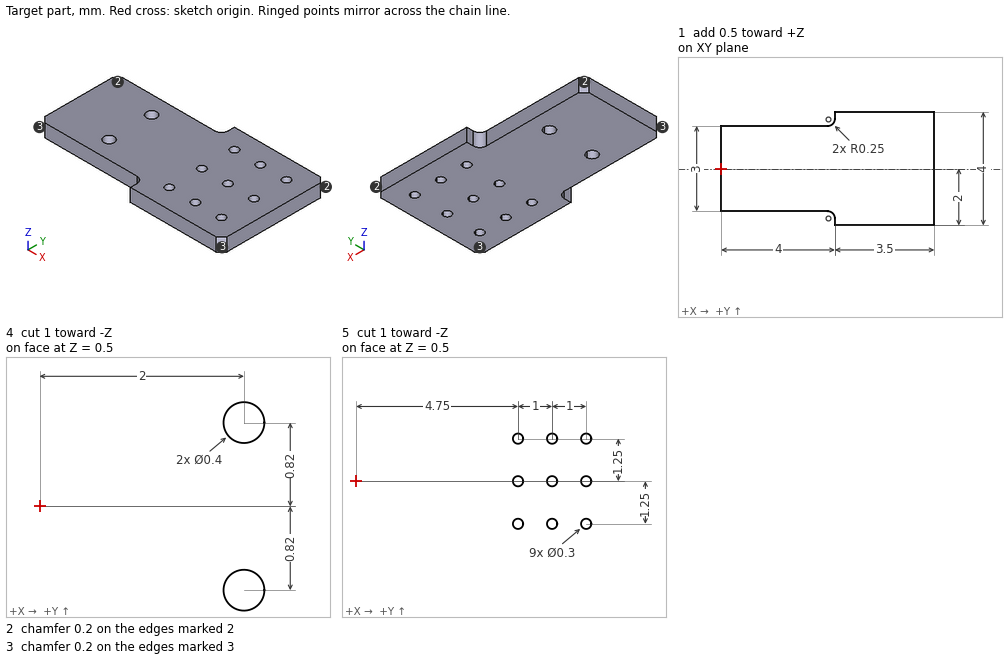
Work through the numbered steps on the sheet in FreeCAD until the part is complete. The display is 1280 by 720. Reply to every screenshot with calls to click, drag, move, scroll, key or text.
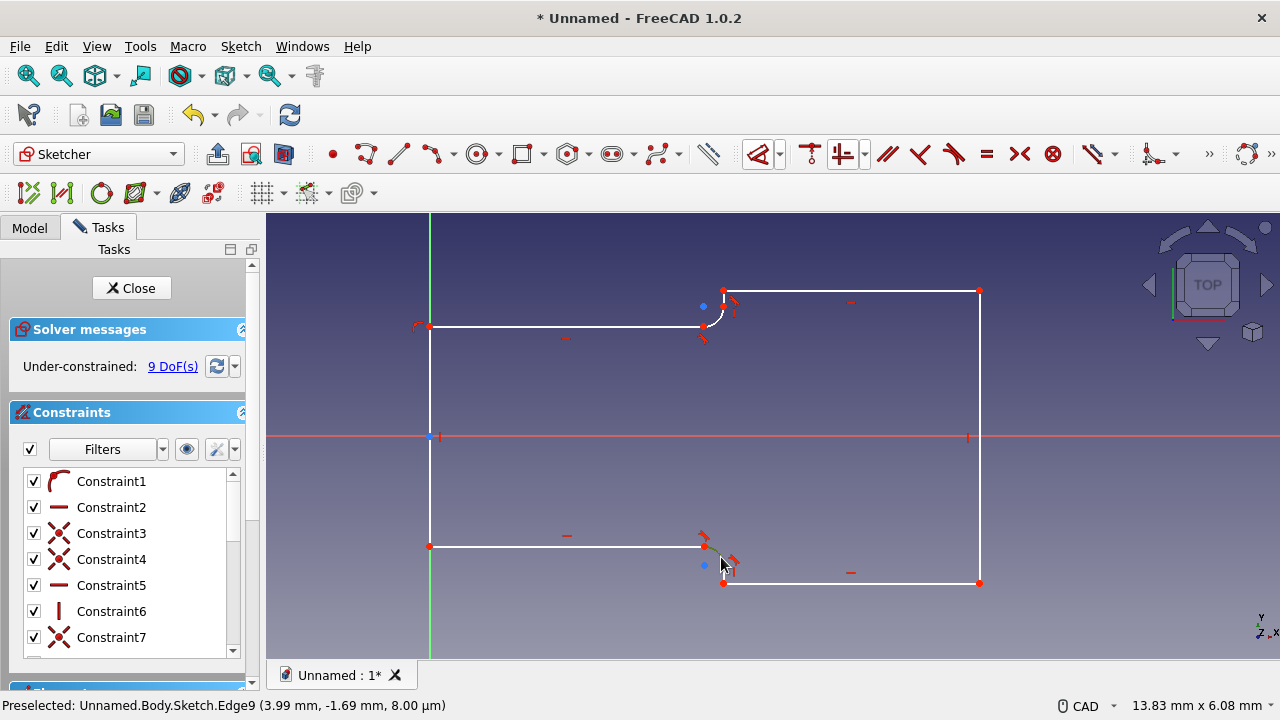
scroll(713, 325, up, 2)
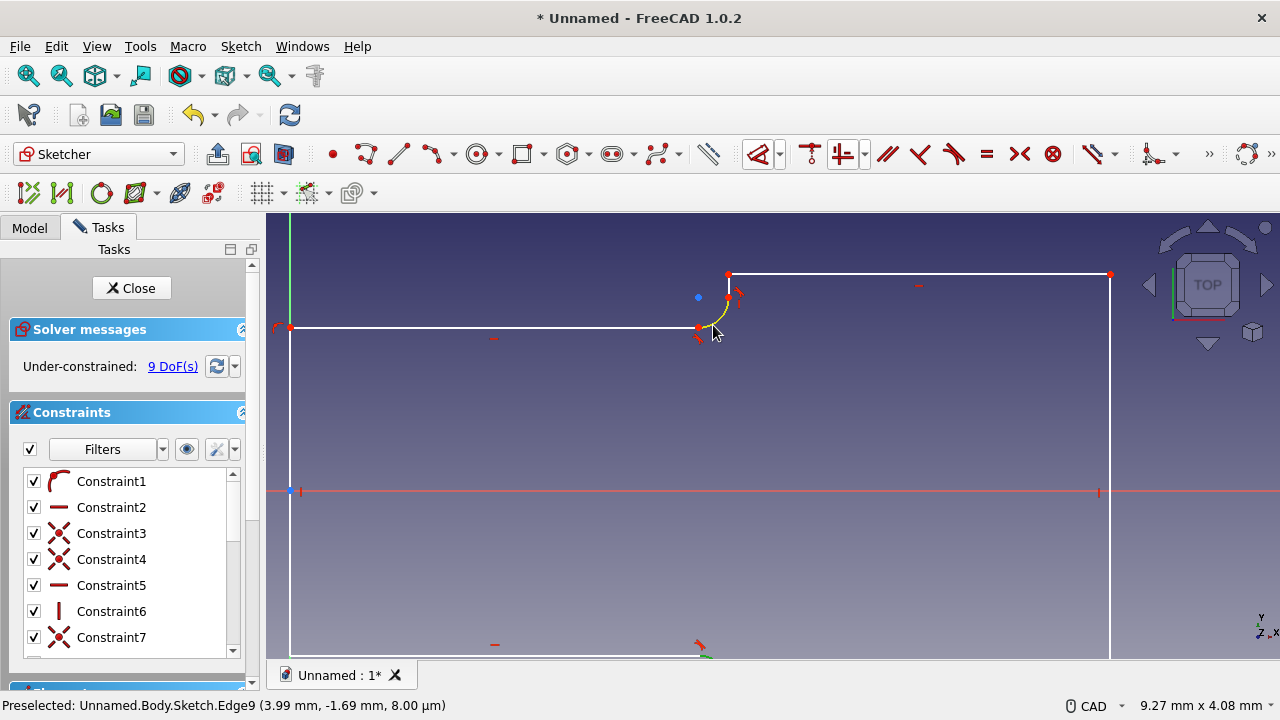
click(712, 325)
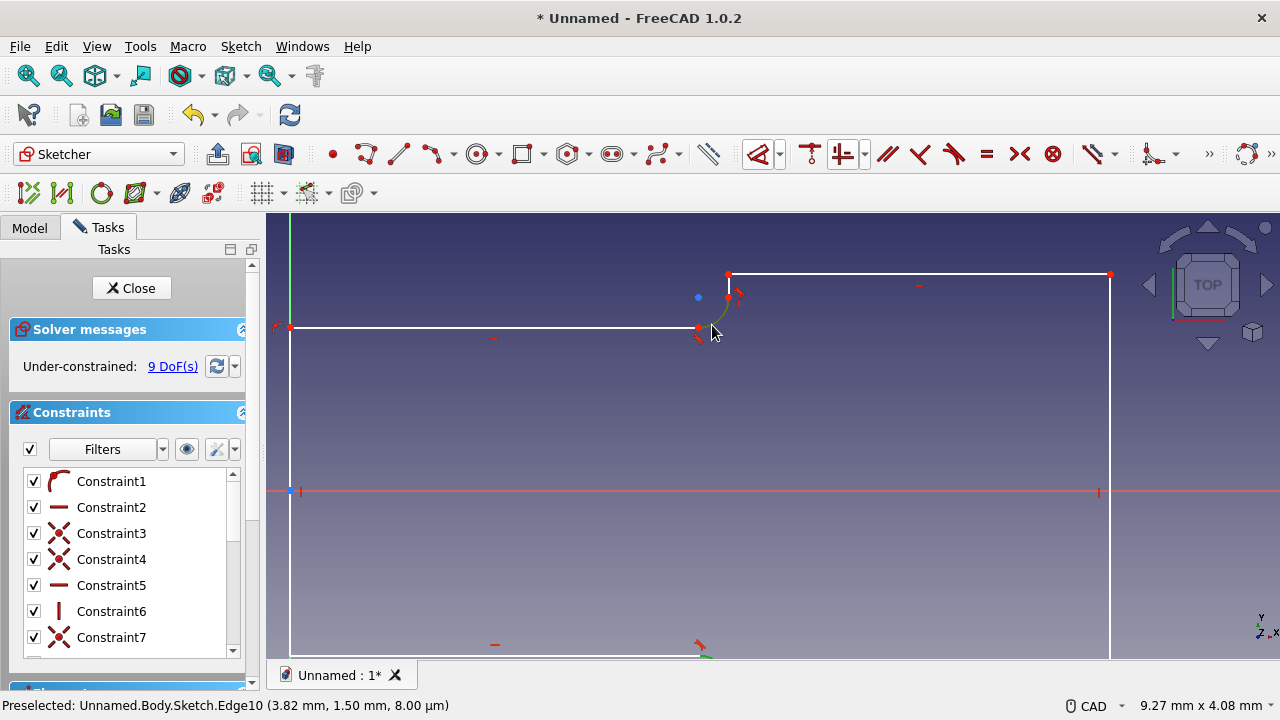
key(e)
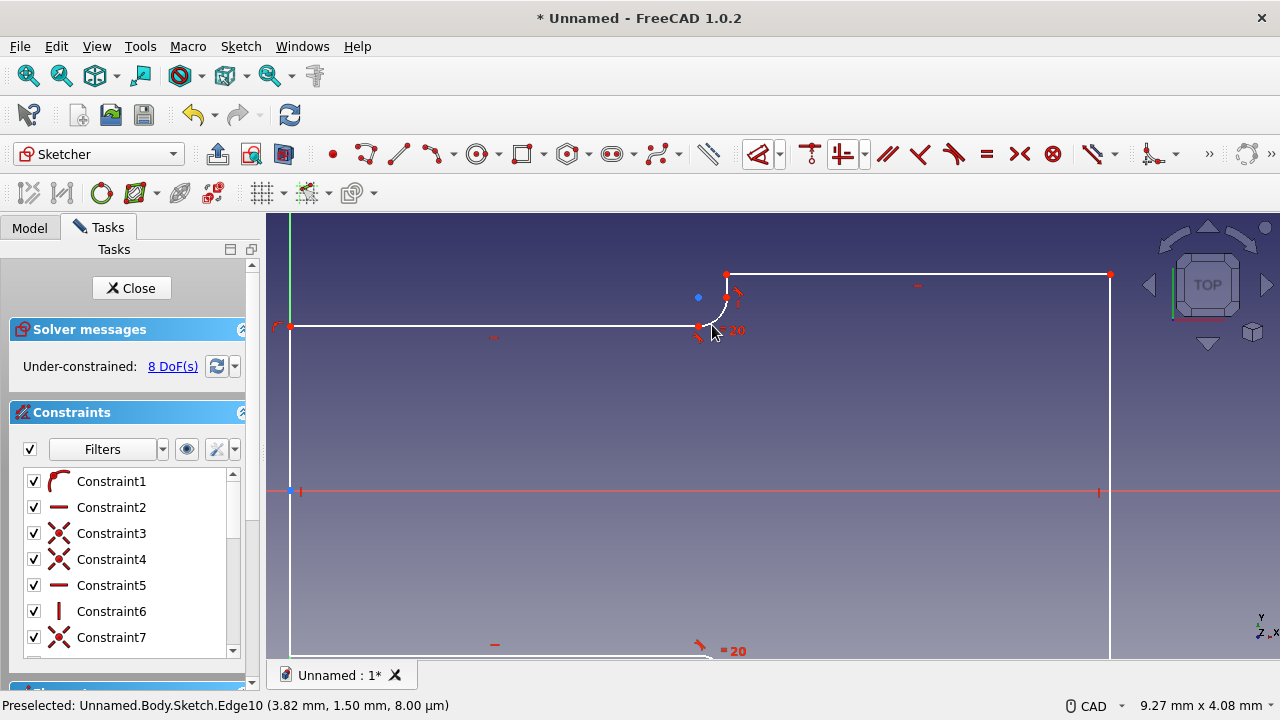
scroll(713, 325, down, 2)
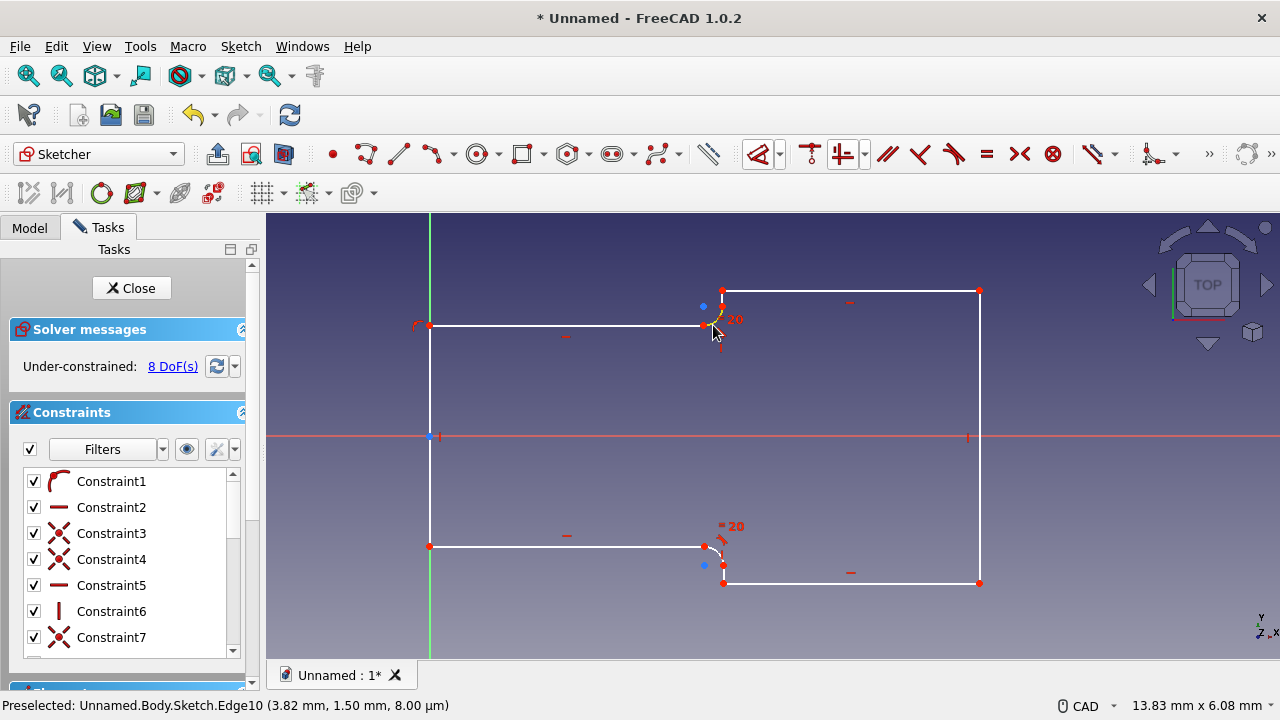
click(705, 566)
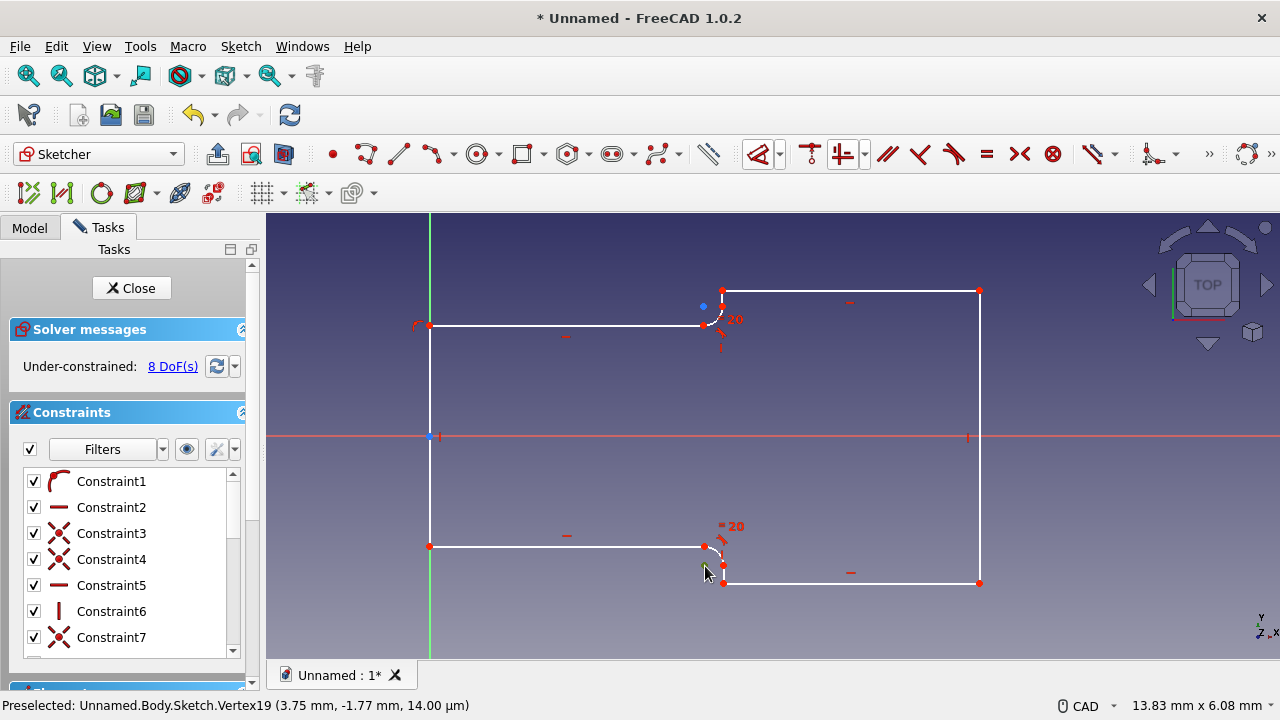
click(703, 307)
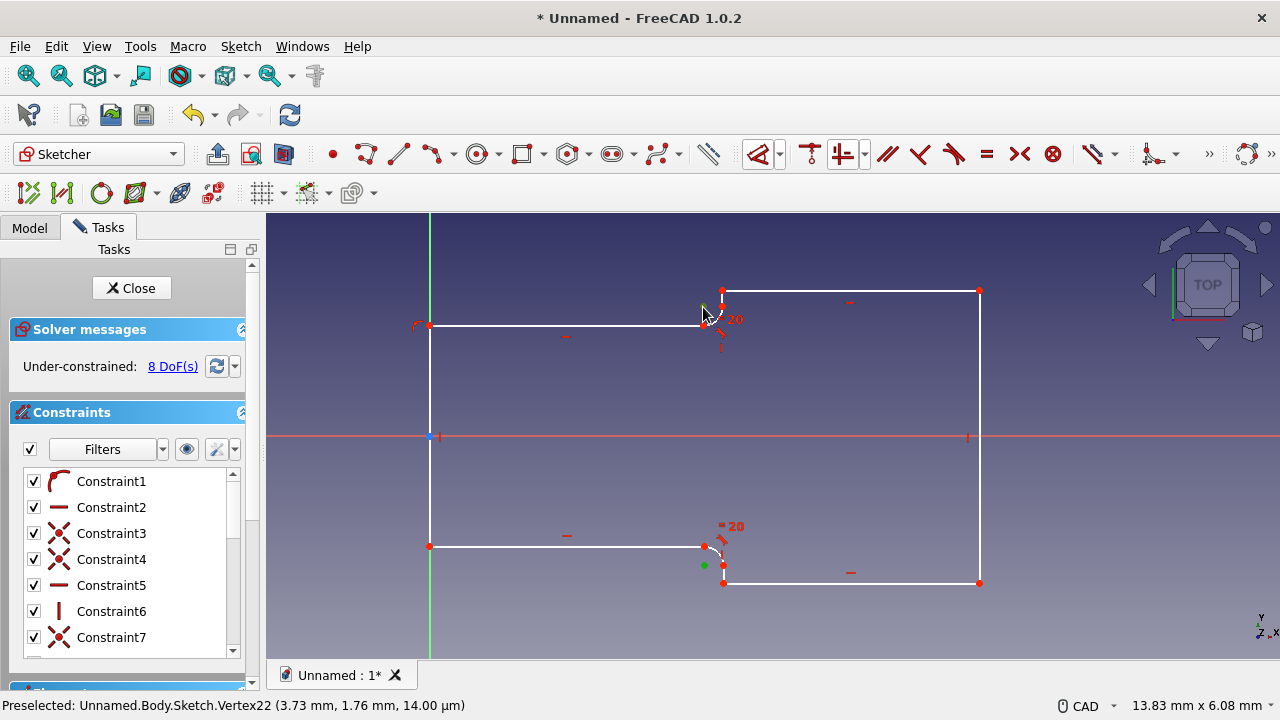
click(353, 436)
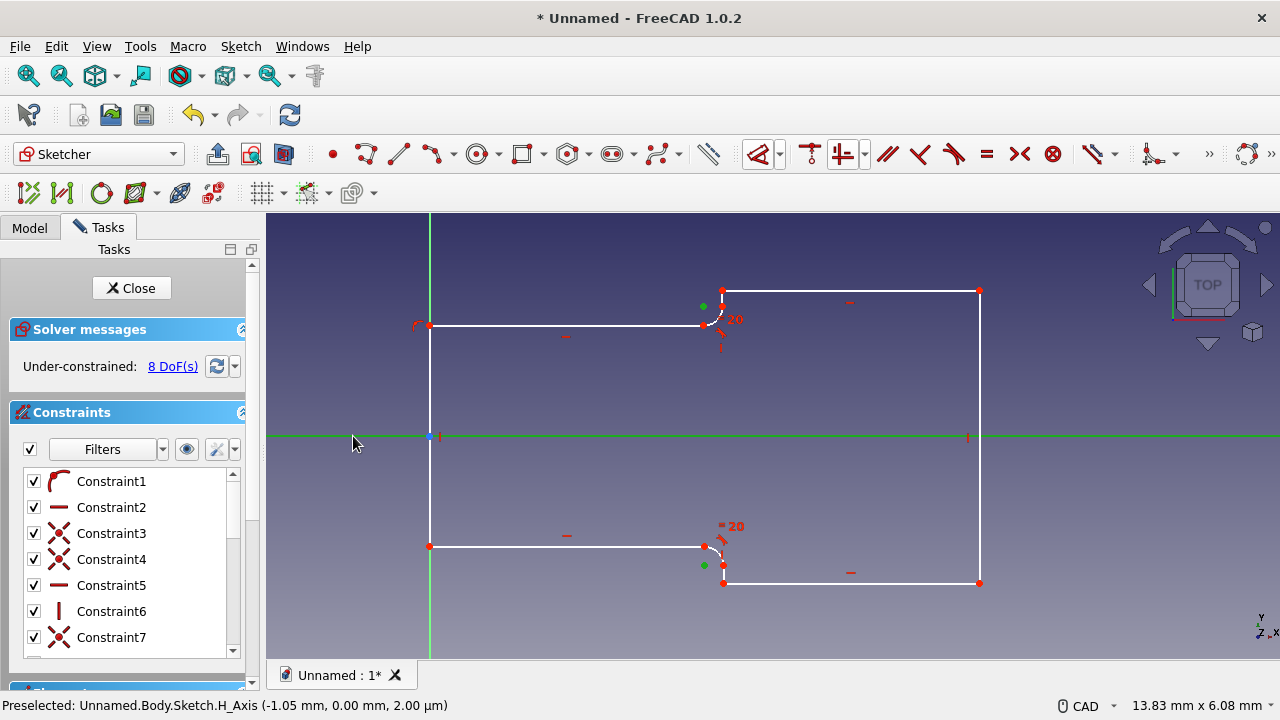
key(s)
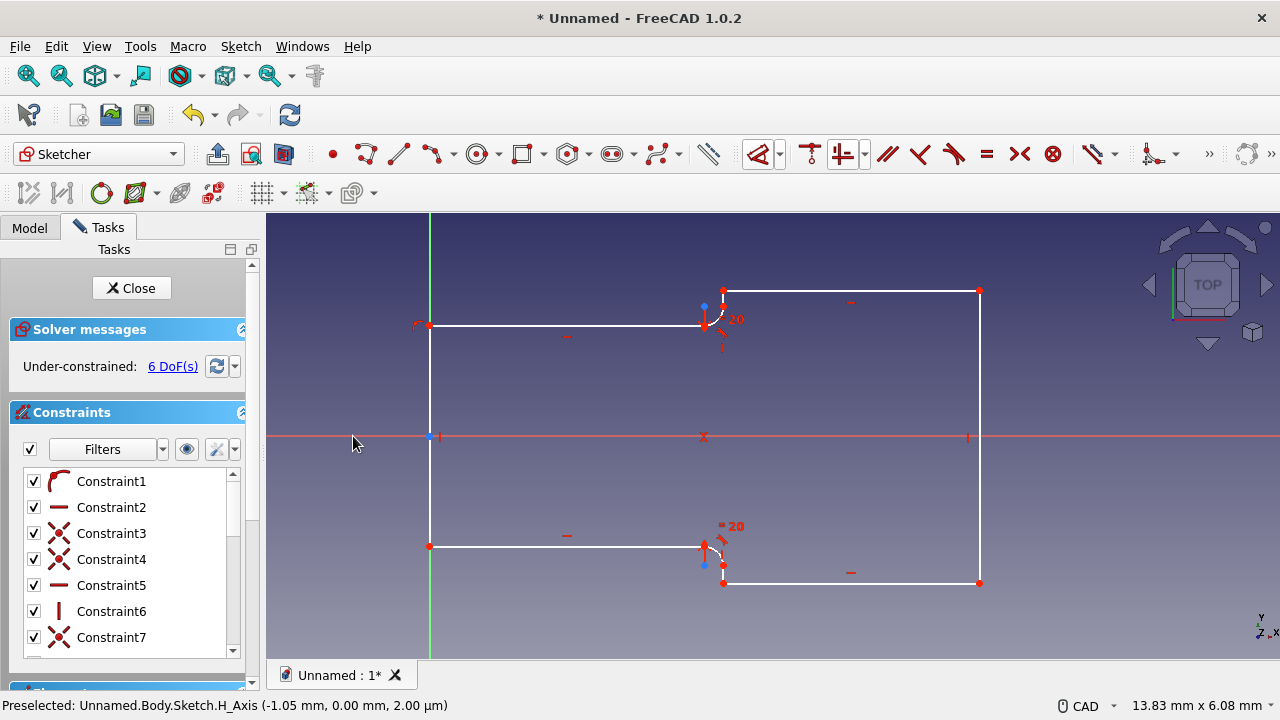
key(d)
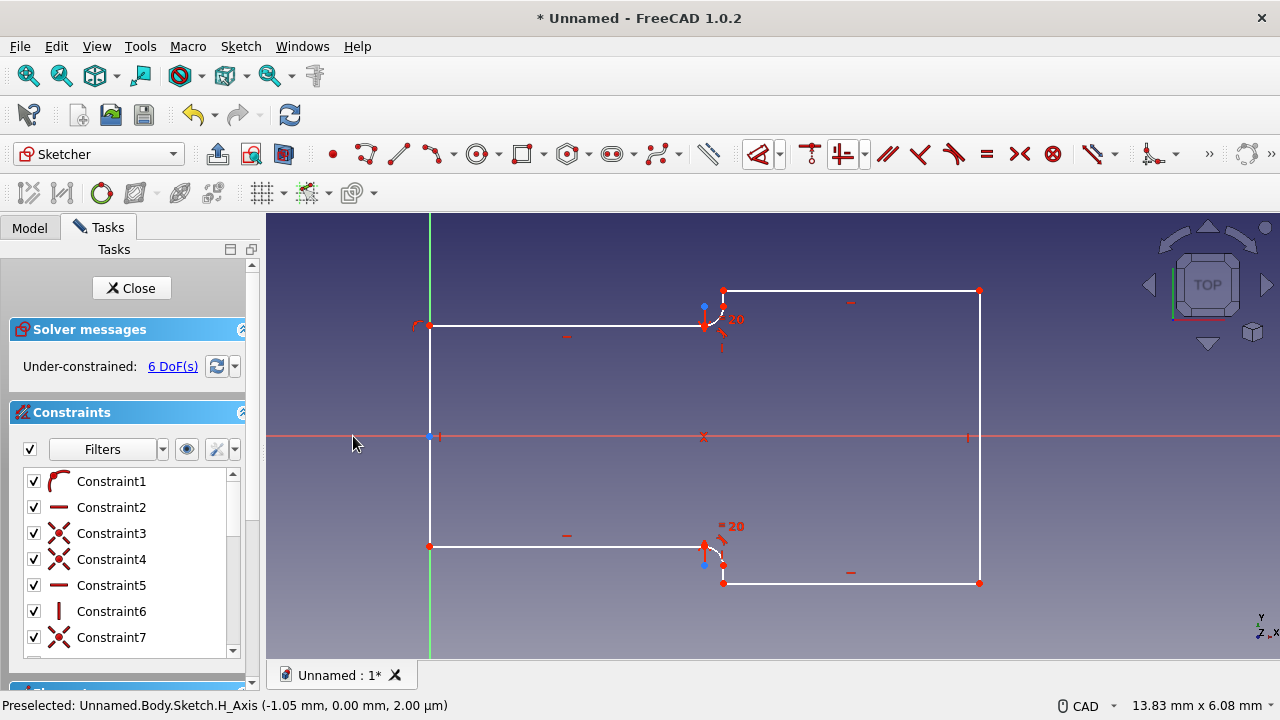
scroll(718, 552, up, 4)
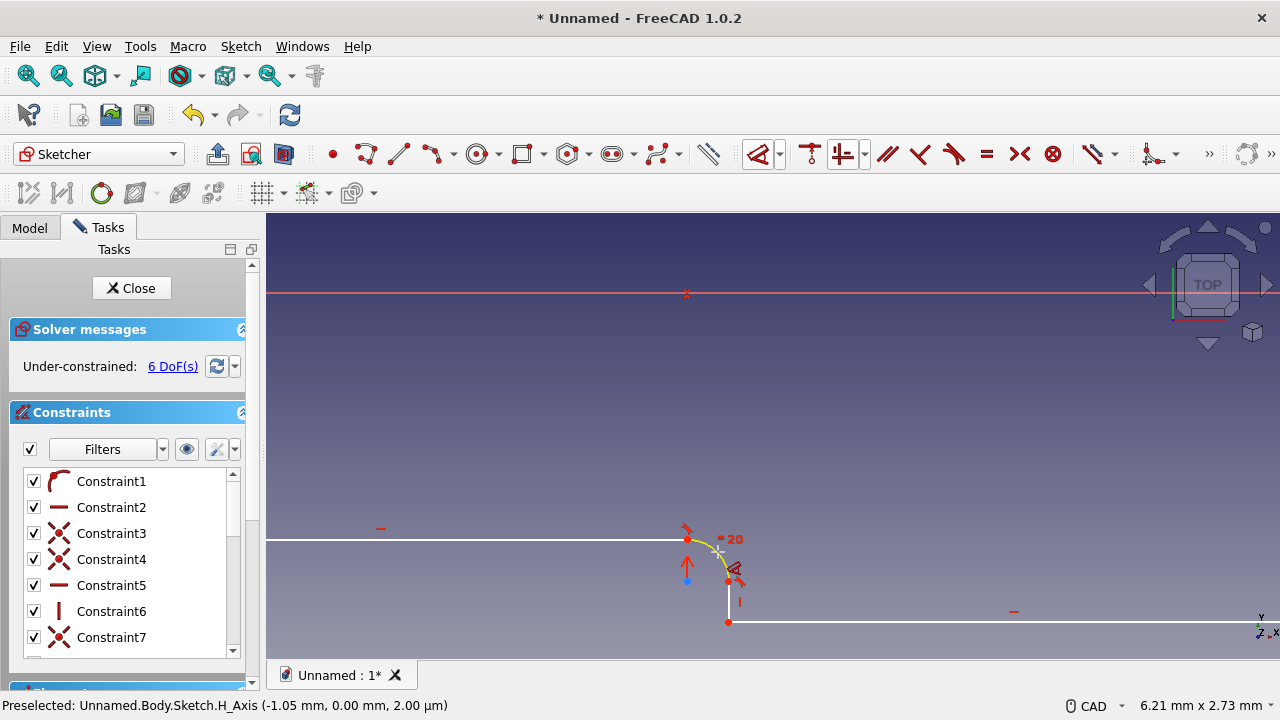
click(717, 552)
click(740, 529)